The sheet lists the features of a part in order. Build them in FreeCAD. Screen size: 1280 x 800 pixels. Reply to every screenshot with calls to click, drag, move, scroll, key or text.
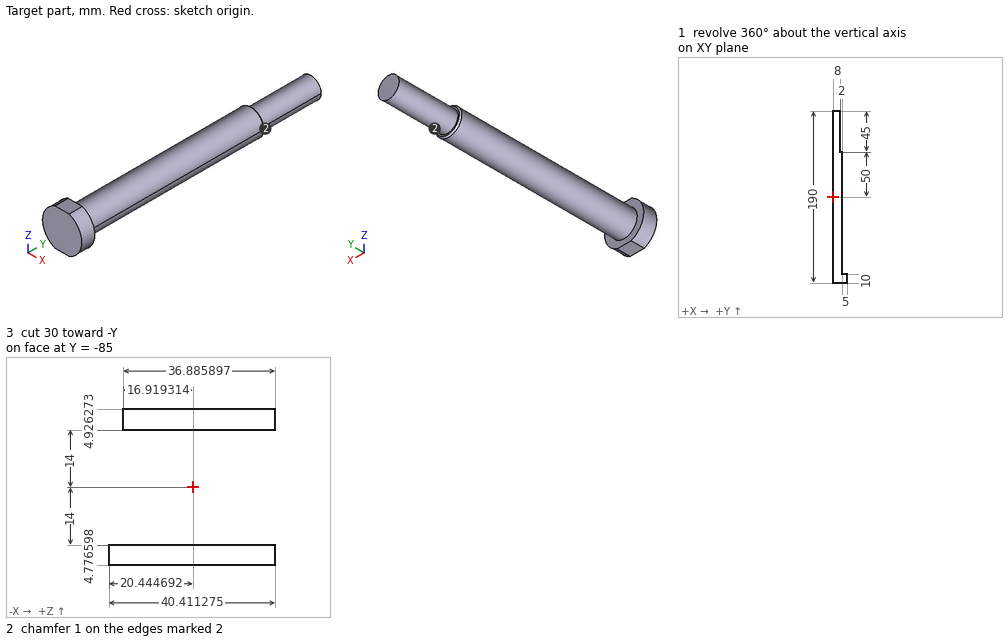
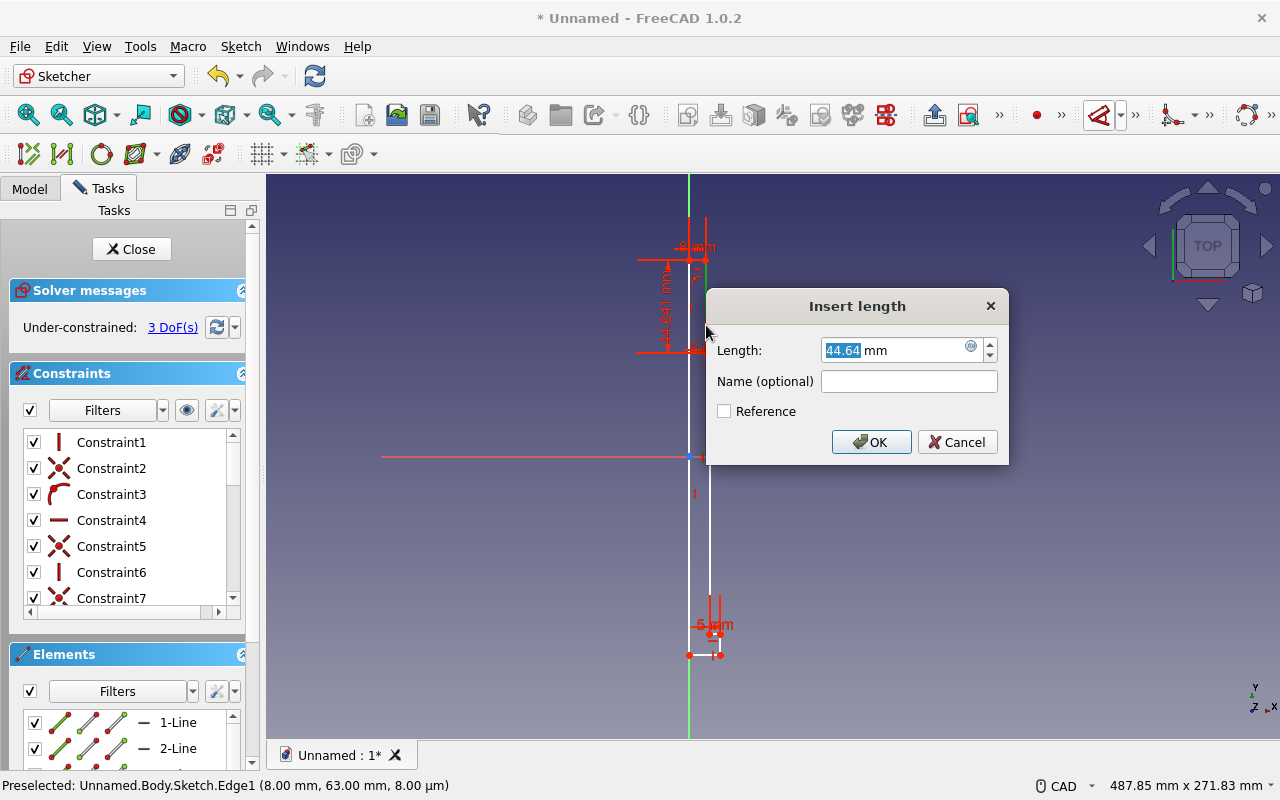
text(45)
key(Return)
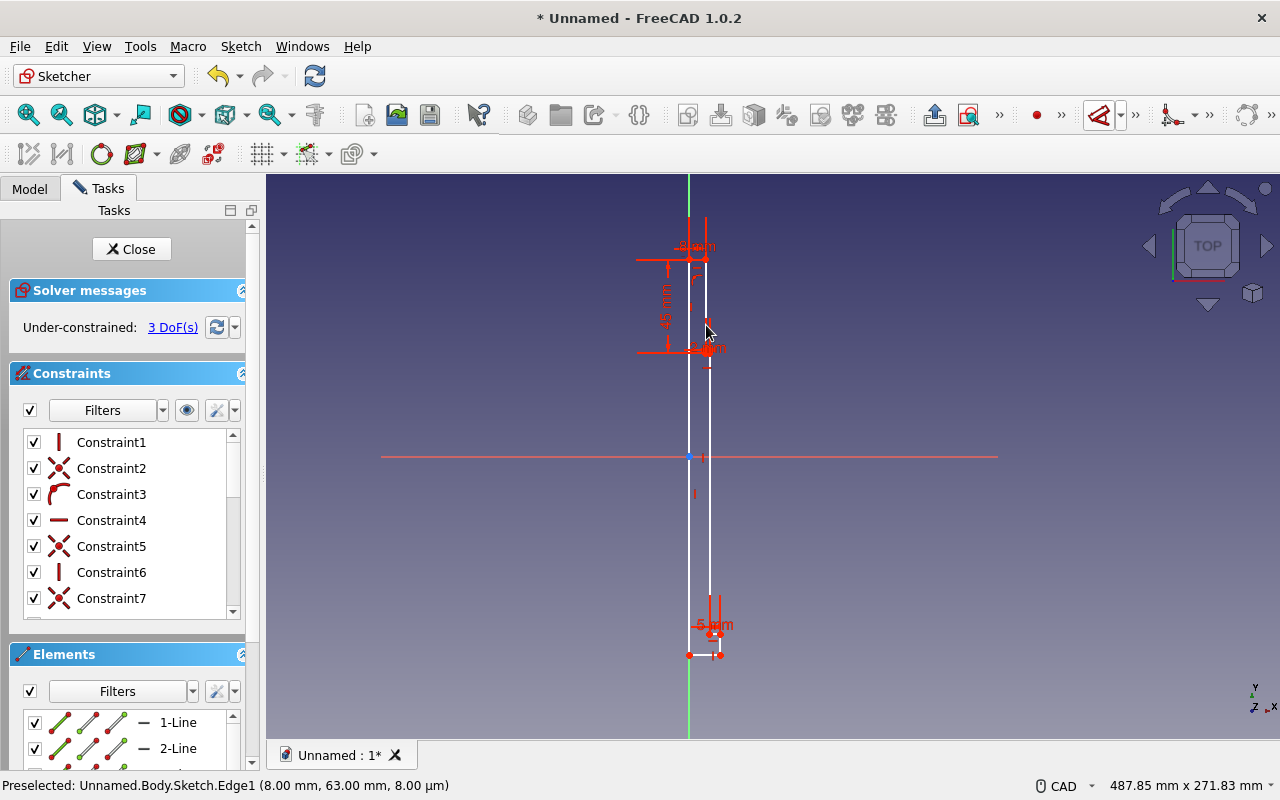
scroll(720, 645, up, 4)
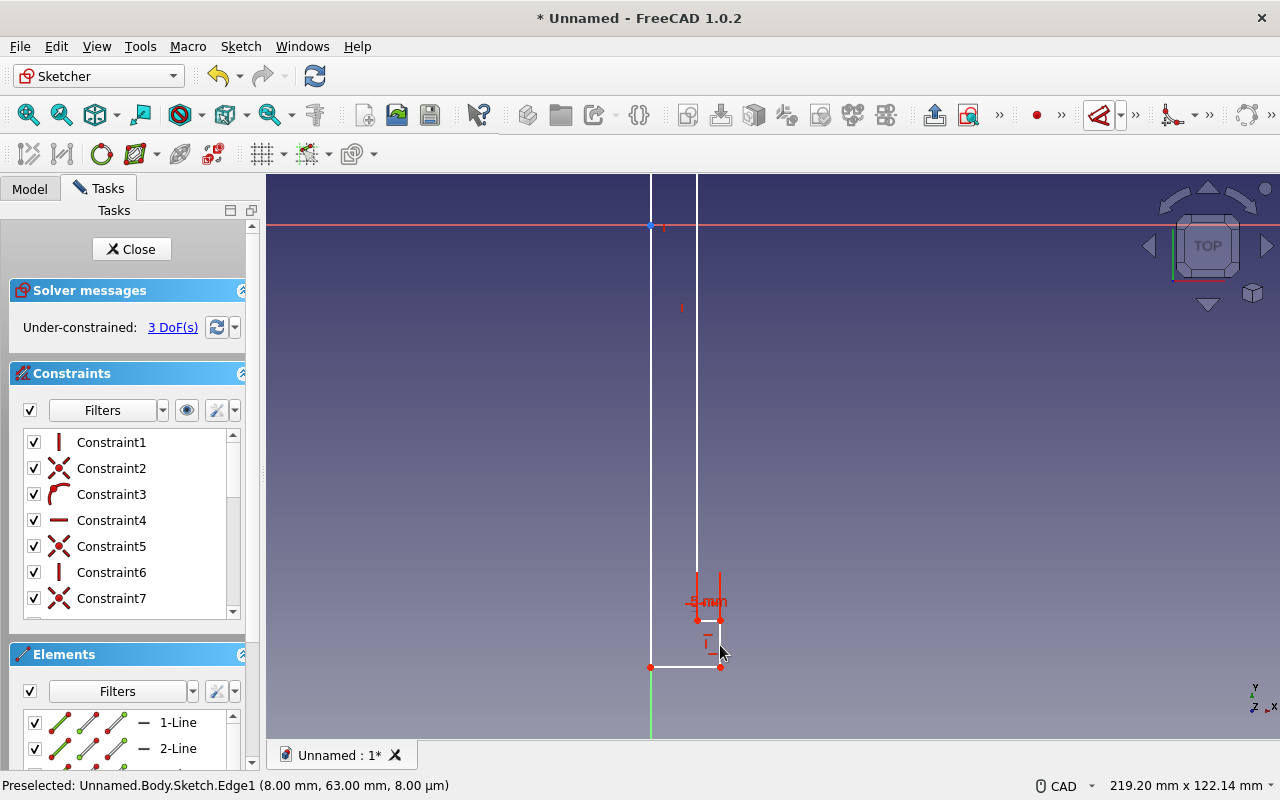
click(720, 644)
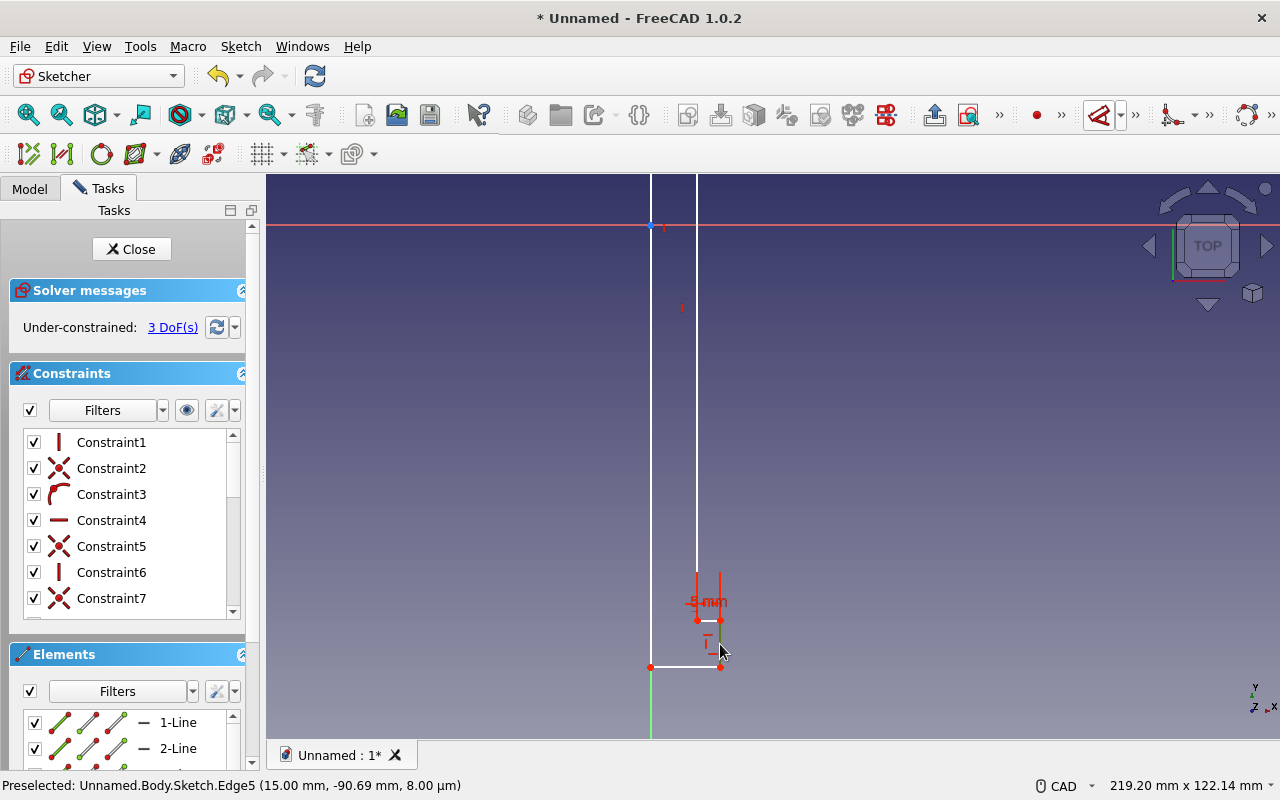
click(1120, 116)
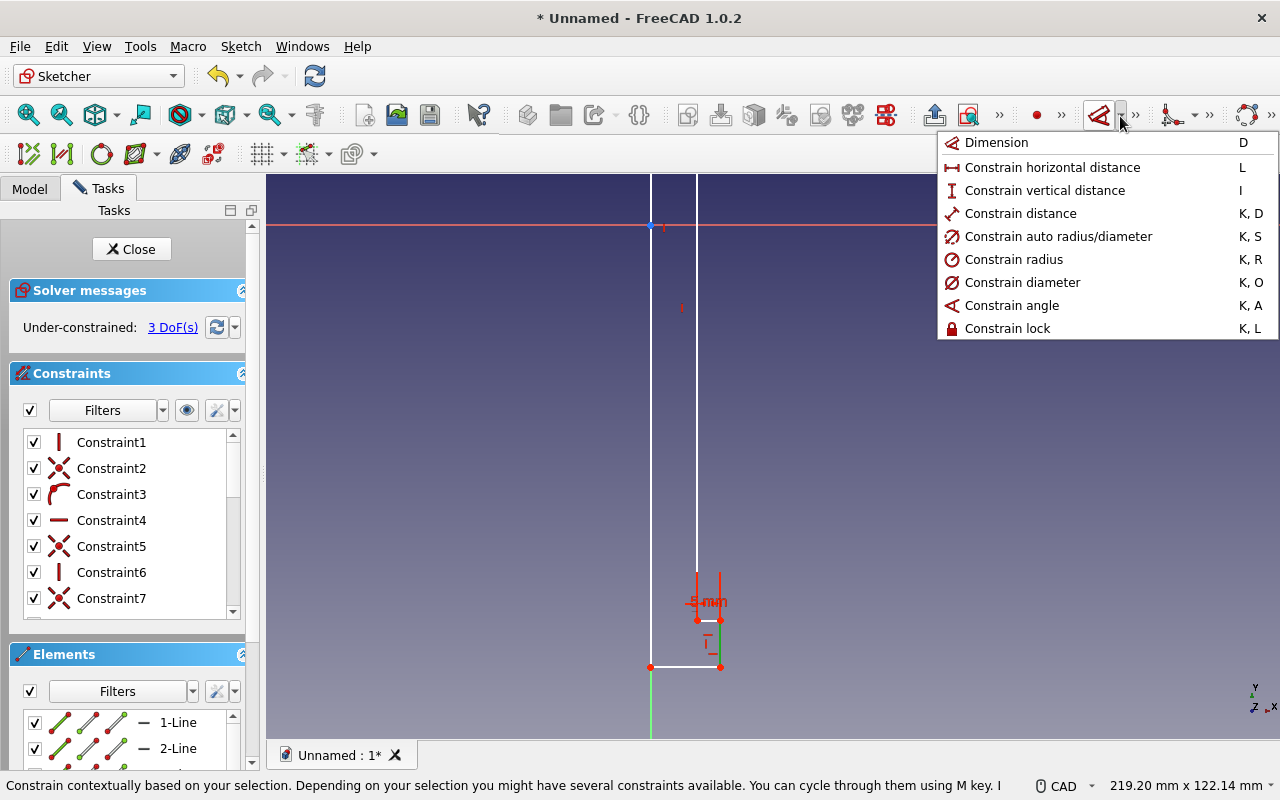
click(1108, 190)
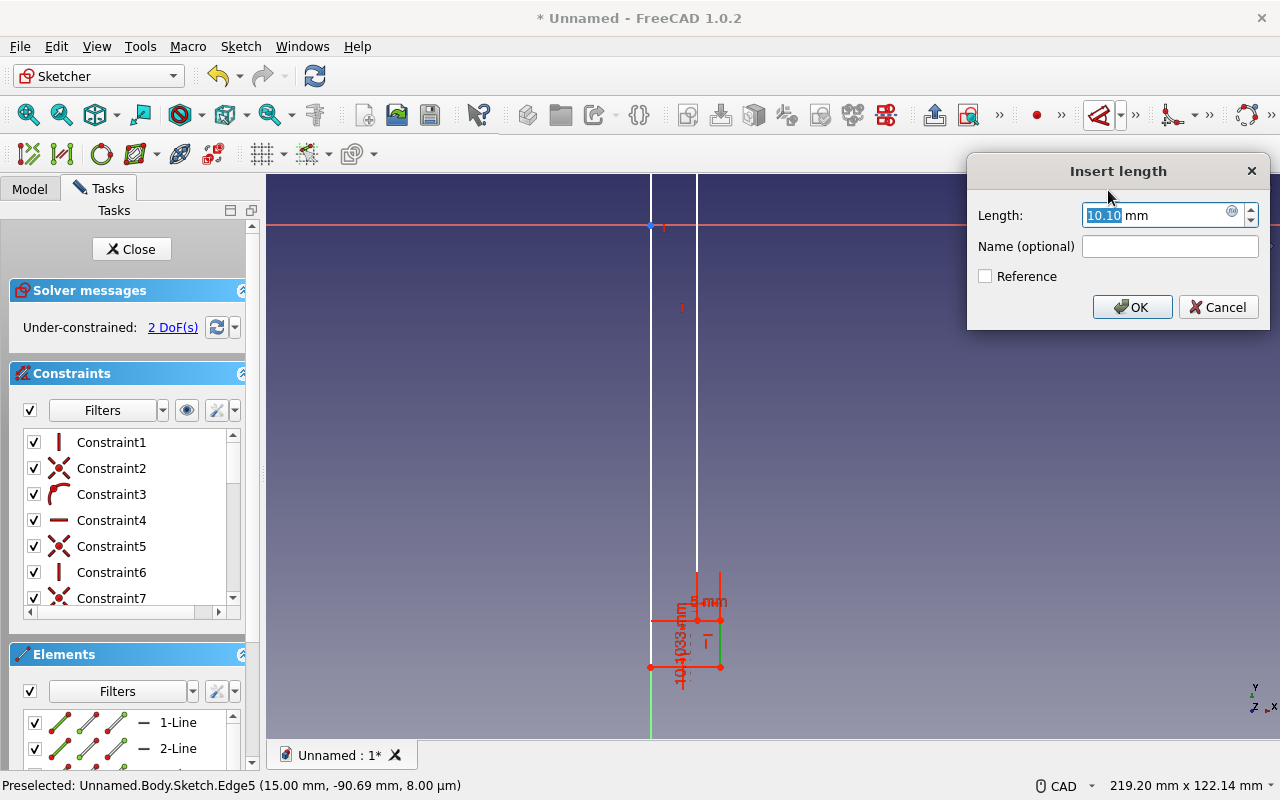
text(10)
key(Return)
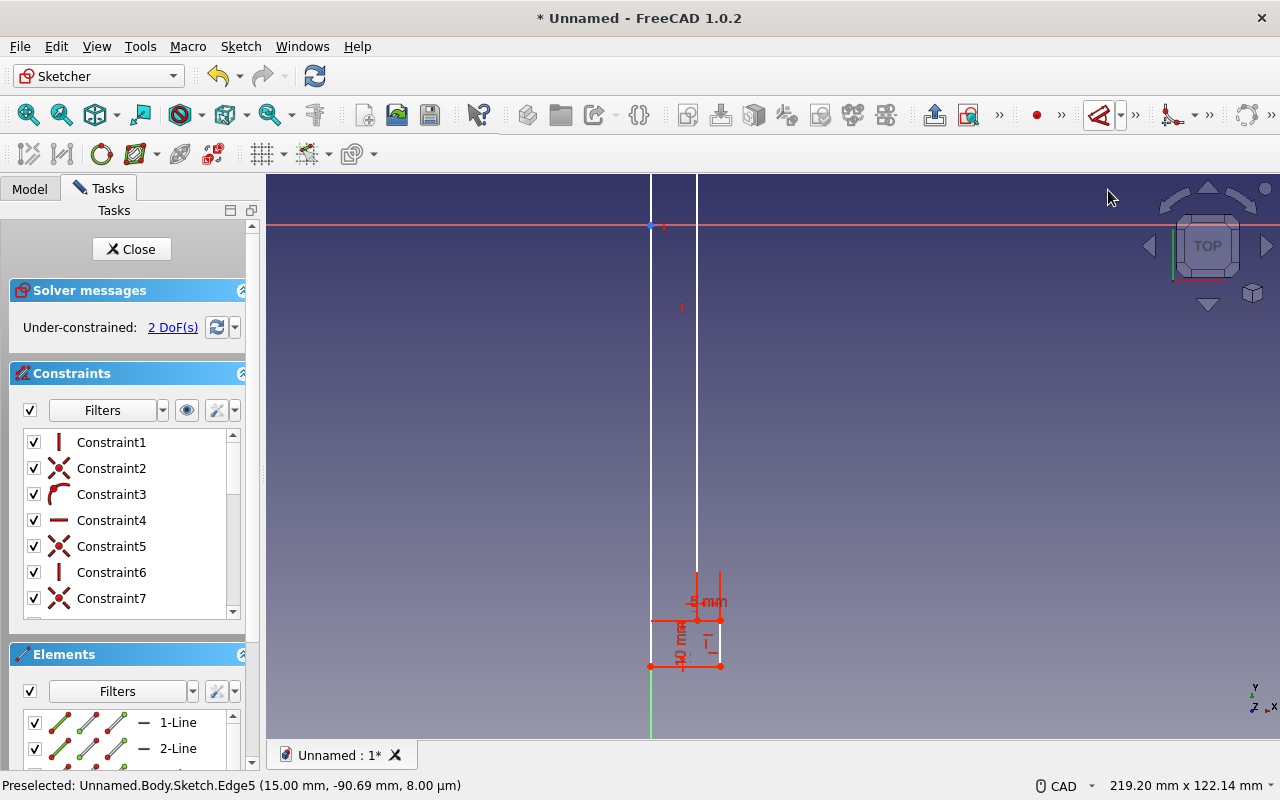
click(651, 403)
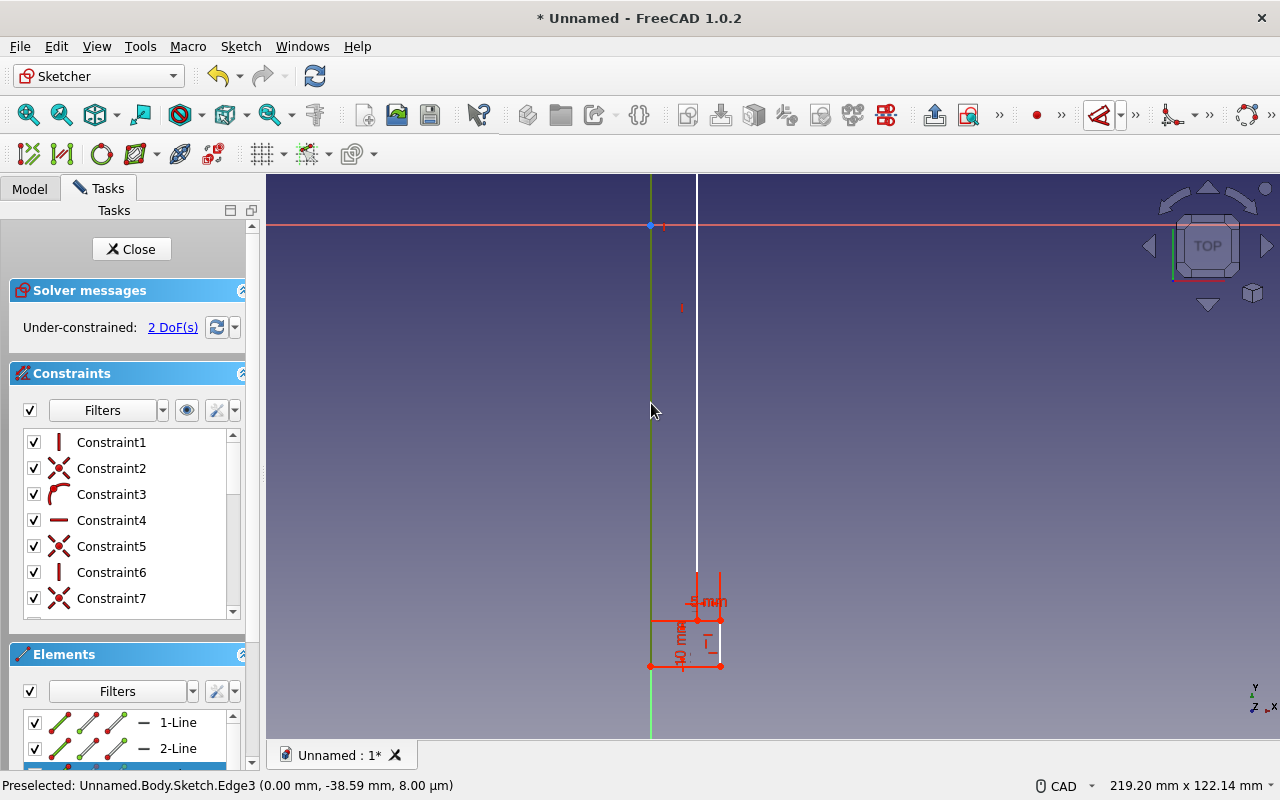
click(1120, 116)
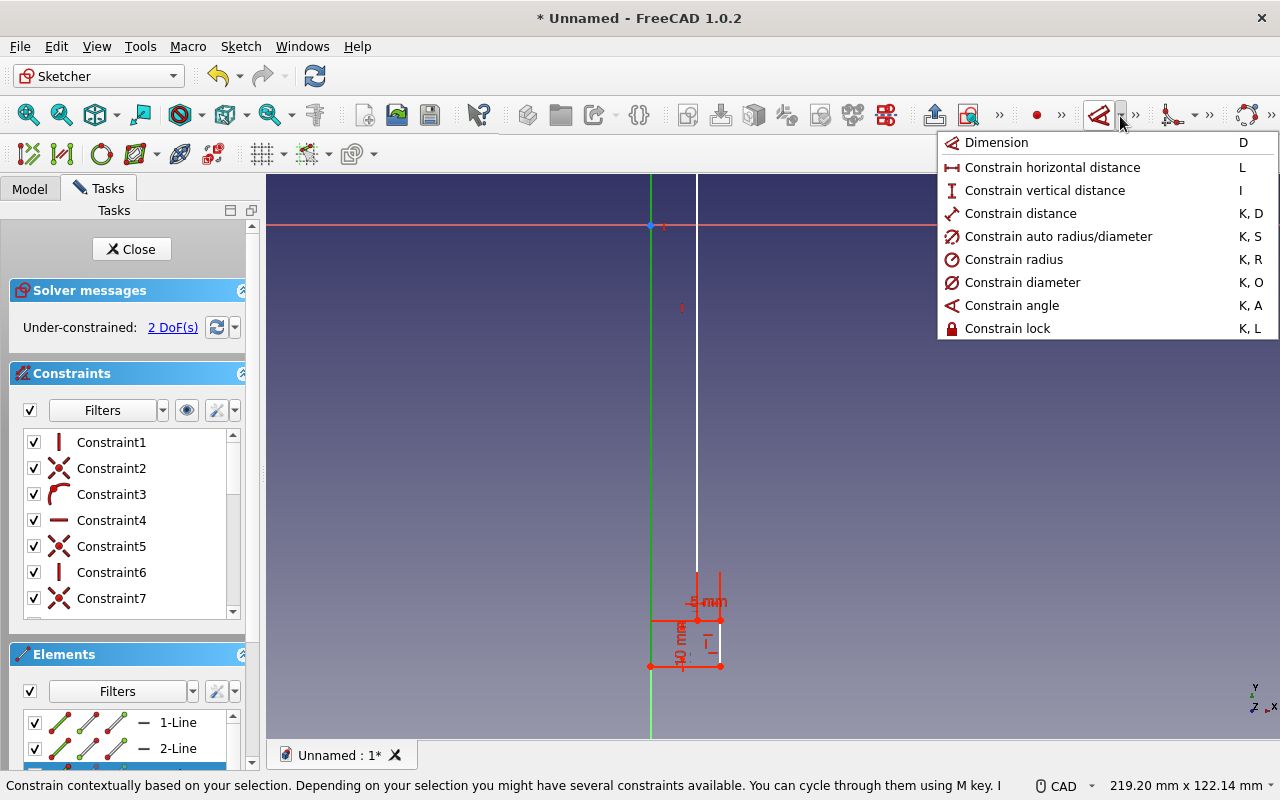
click(1108, 190)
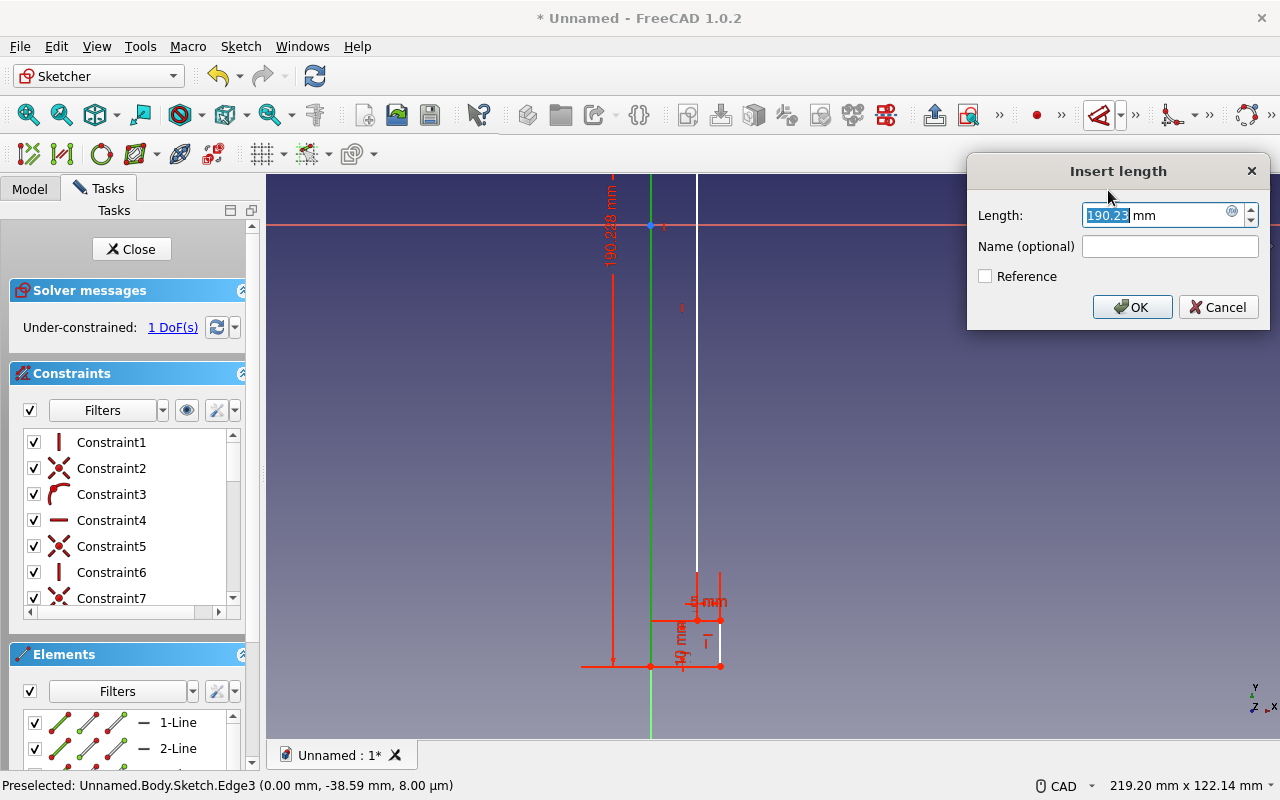
text(190)
key(Return)